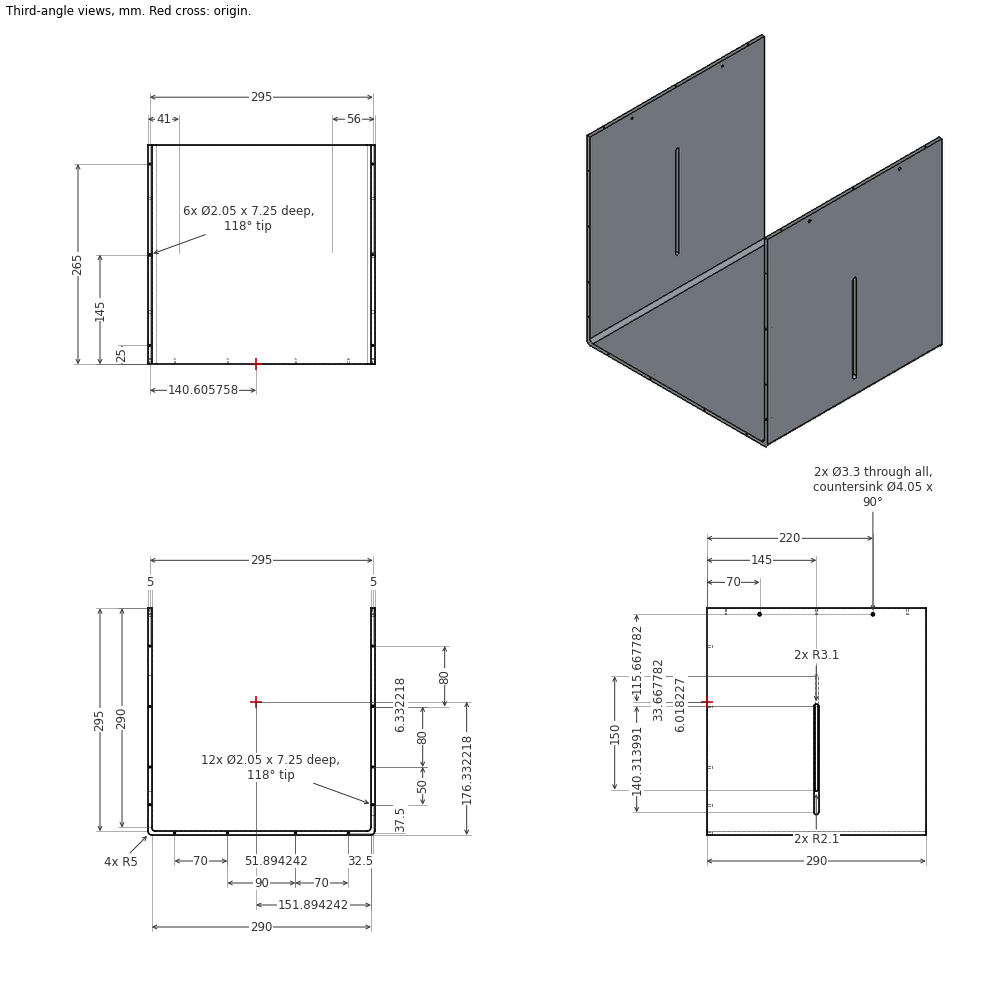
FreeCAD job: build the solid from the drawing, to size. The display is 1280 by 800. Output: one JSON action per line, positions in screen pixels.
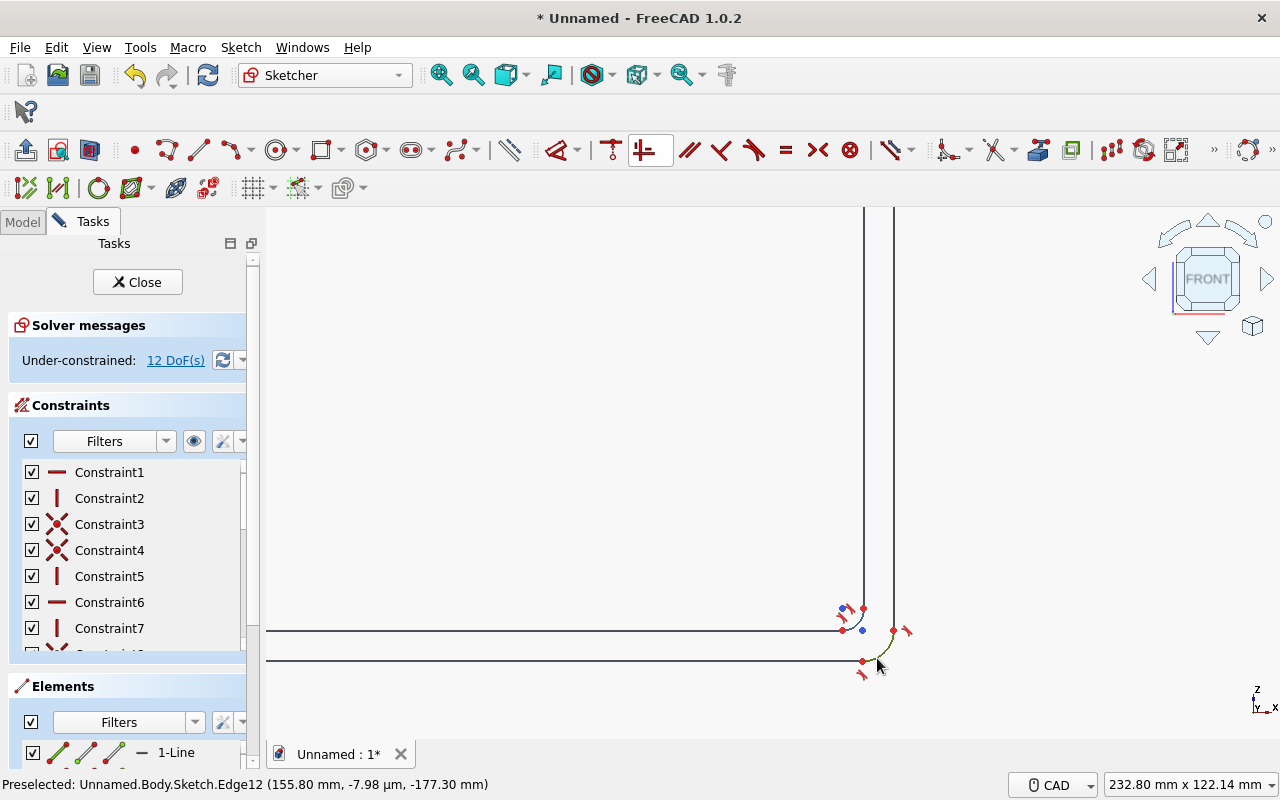
{"action": "left_click", "coordinate": [786, 150]}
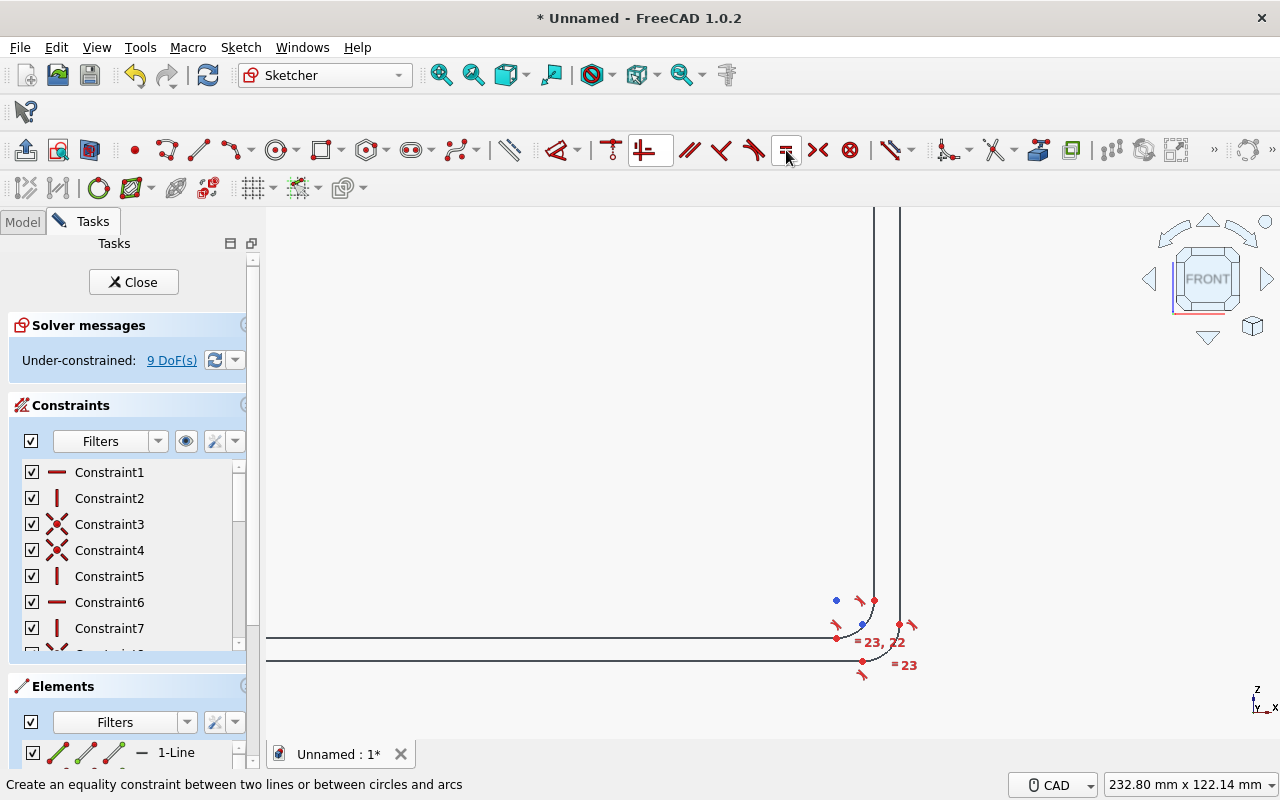
{"action": "left_click", "coordinate": [556, 150]}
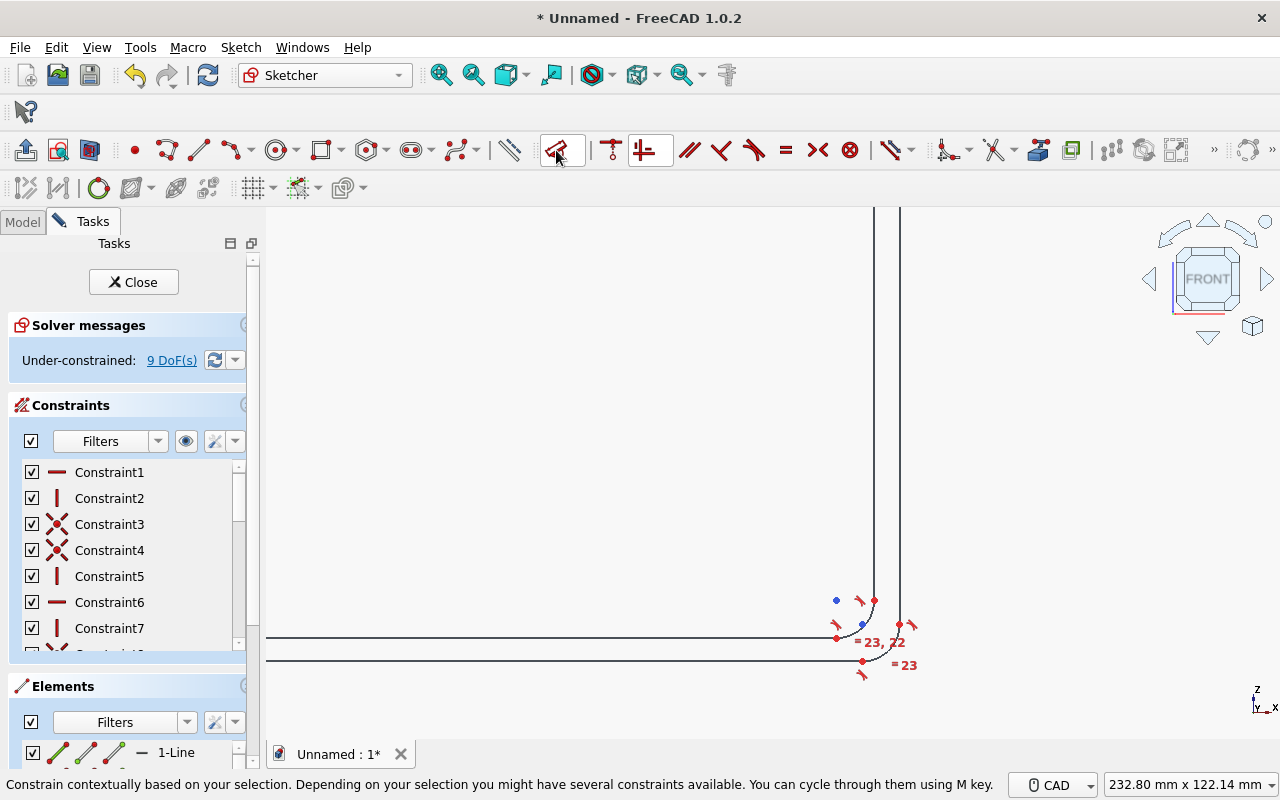
{"action": "scroll", "coordinate": [859, 628], "scroll_direction": "down", "scroll_amount": 7}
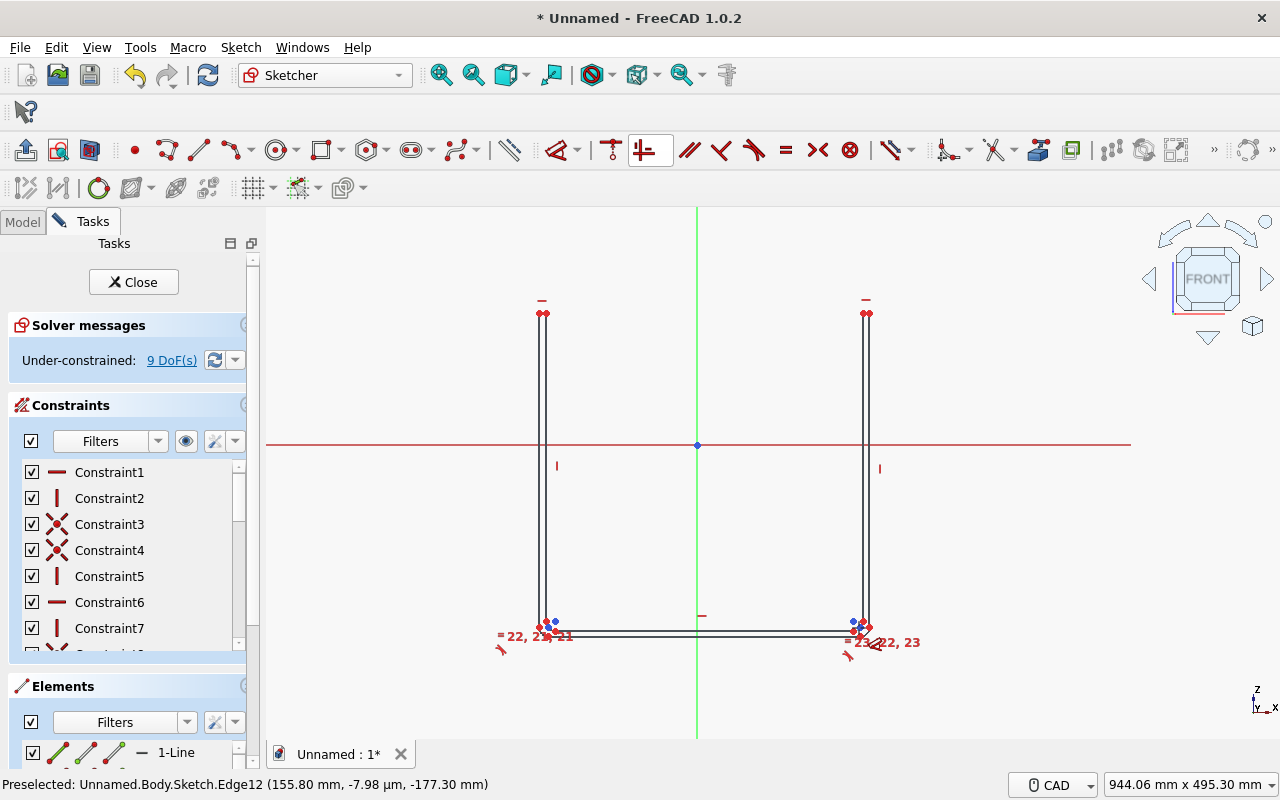
{"action": "scroll", "coordinate": [540, 632], "scroll_direction": "up", "scroll_amount": 11}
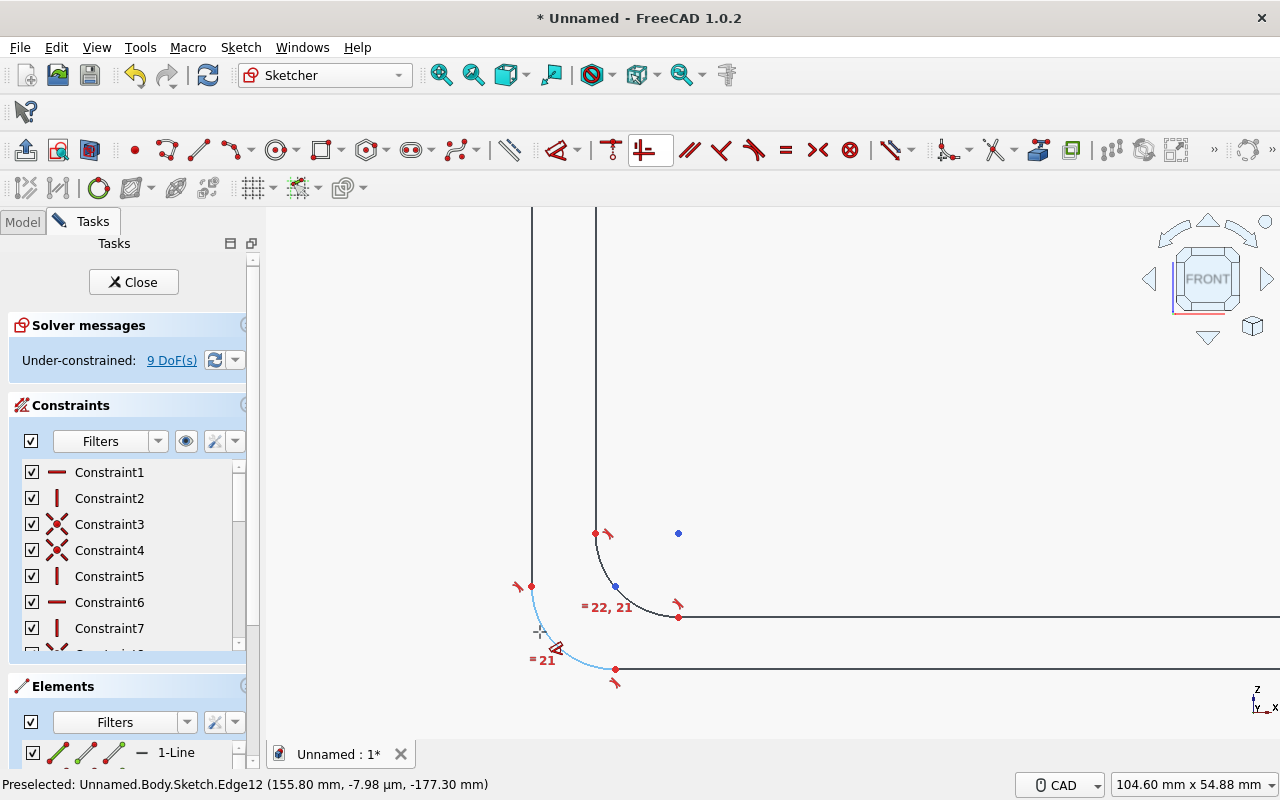
{"action": "left_click", "coordinate": [541, 624]}
{"action": "left_click", "coordinate": [513, 639]}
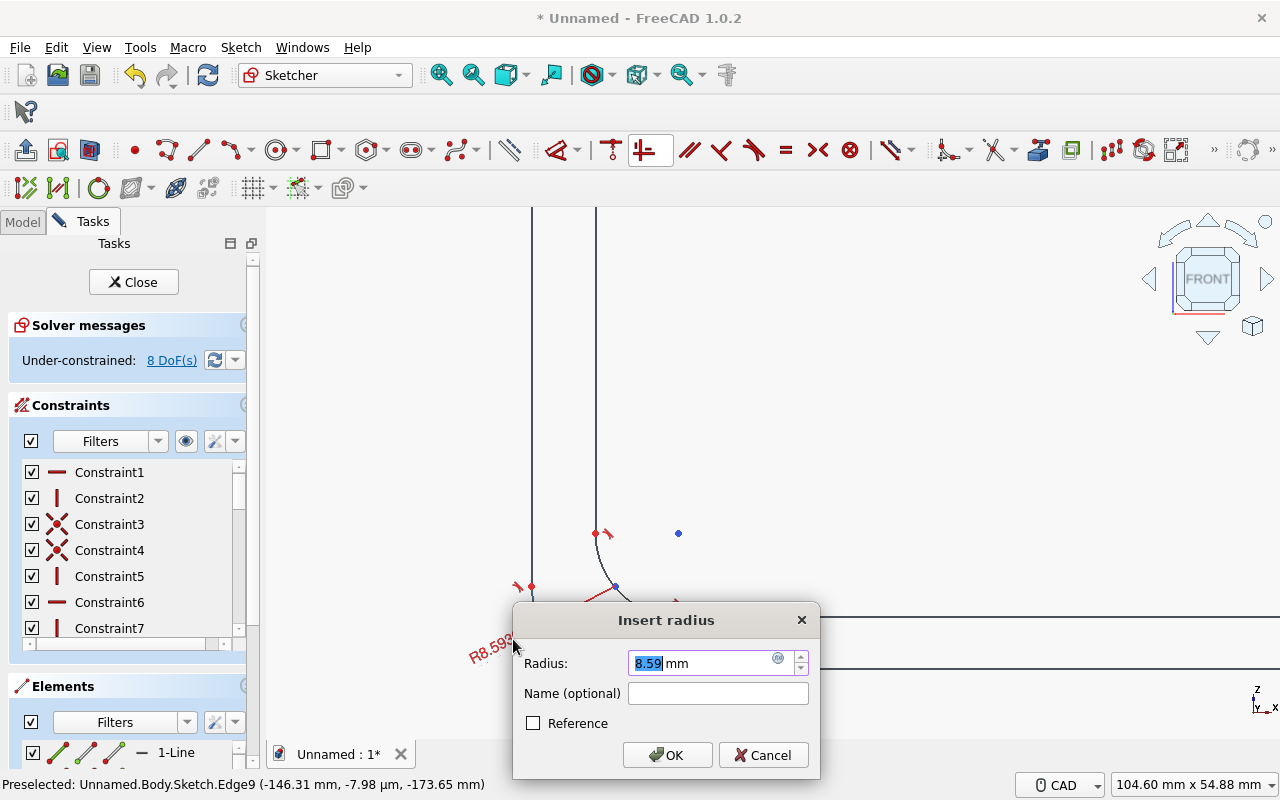
{"action": "type", "text": "5"}
{"action": "key", "text": "Return"}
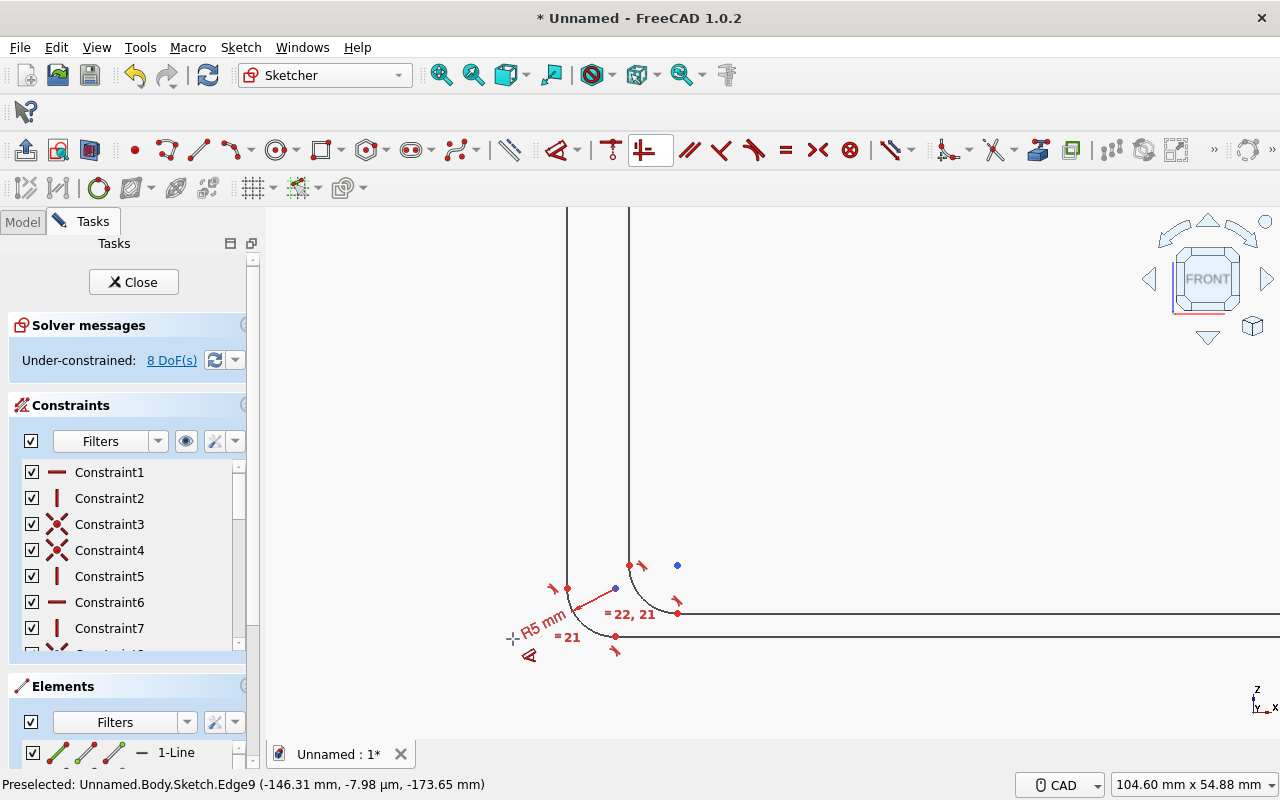
{"action": "scroll", "coordinate": [540, 632], "scroll_direction": "down", "scroll_amount": 11}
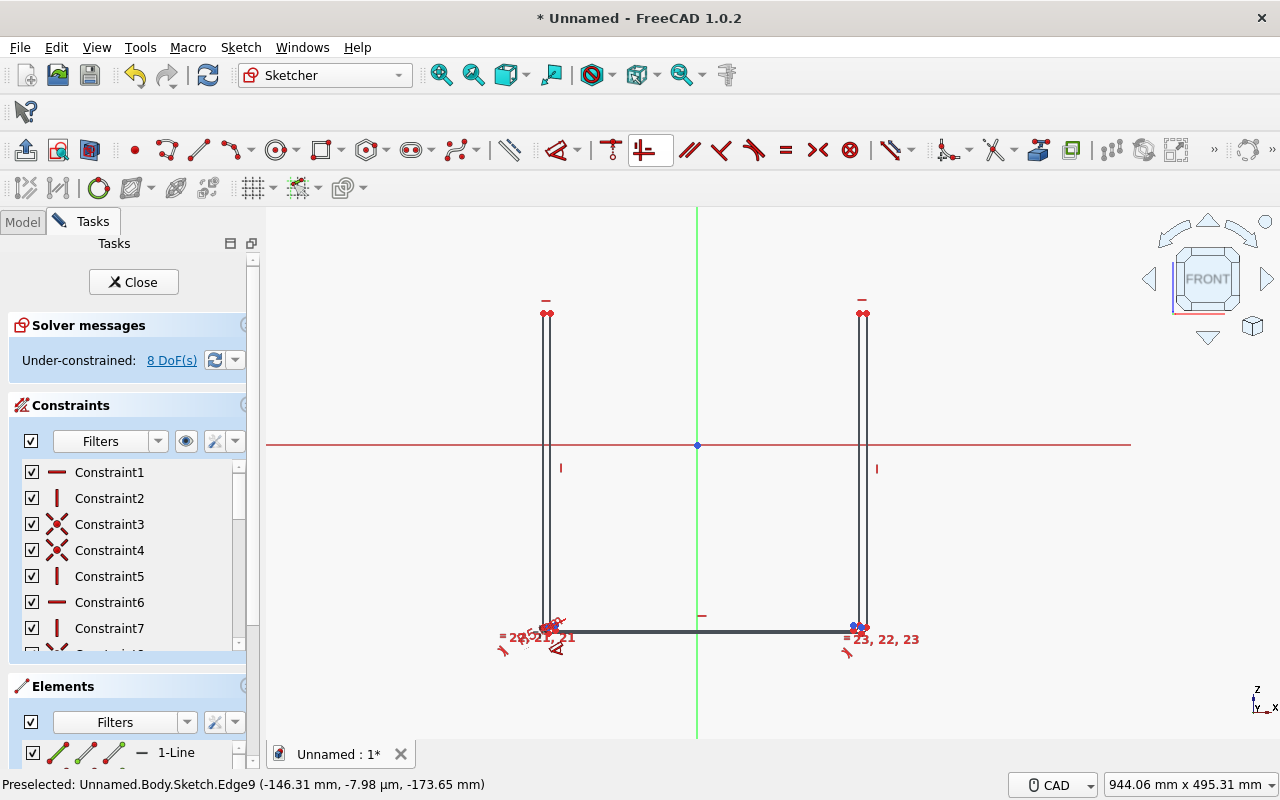
{"action": "scroll", "coordinate": [545, 314], "scroll_direction": "up", "scroll_amount": 11}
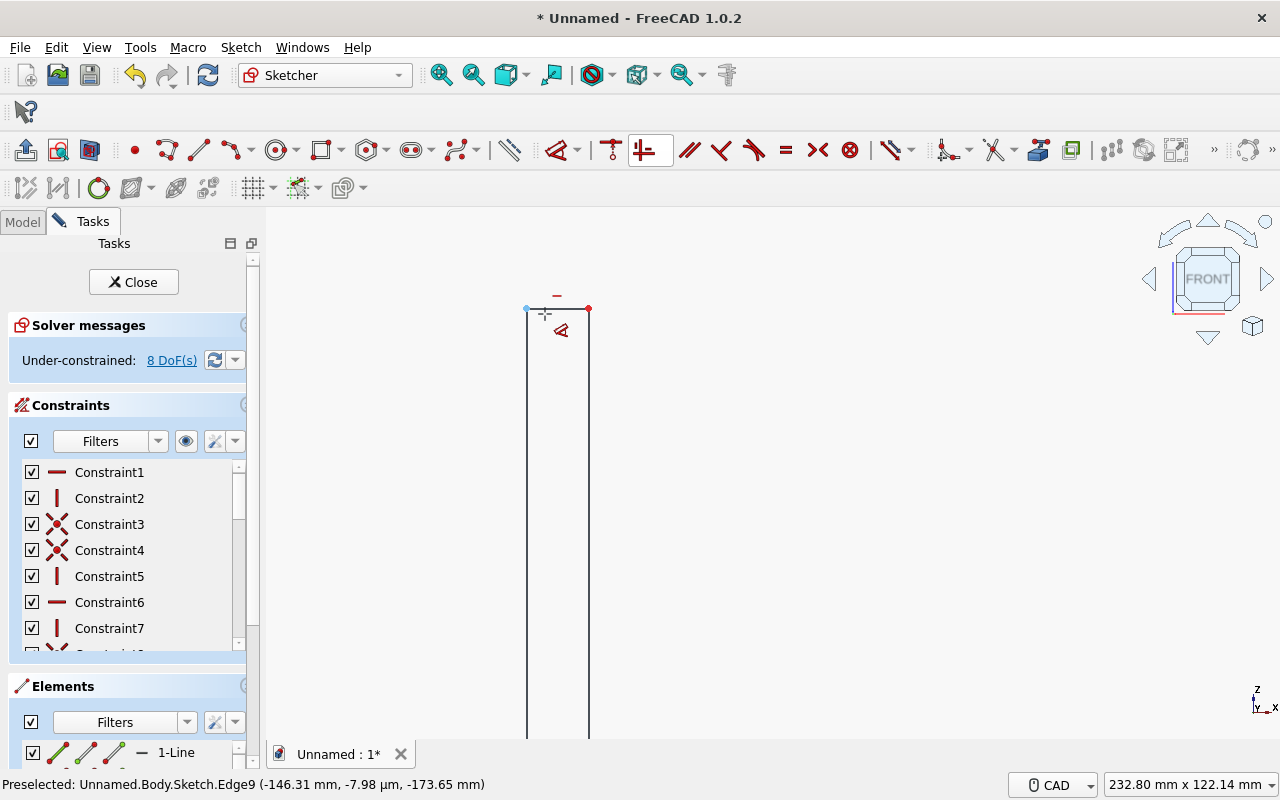
{"action": "left_click", "coordinate": [546, 309]}
{"action": "left_click", "coordinate": [558, 275]}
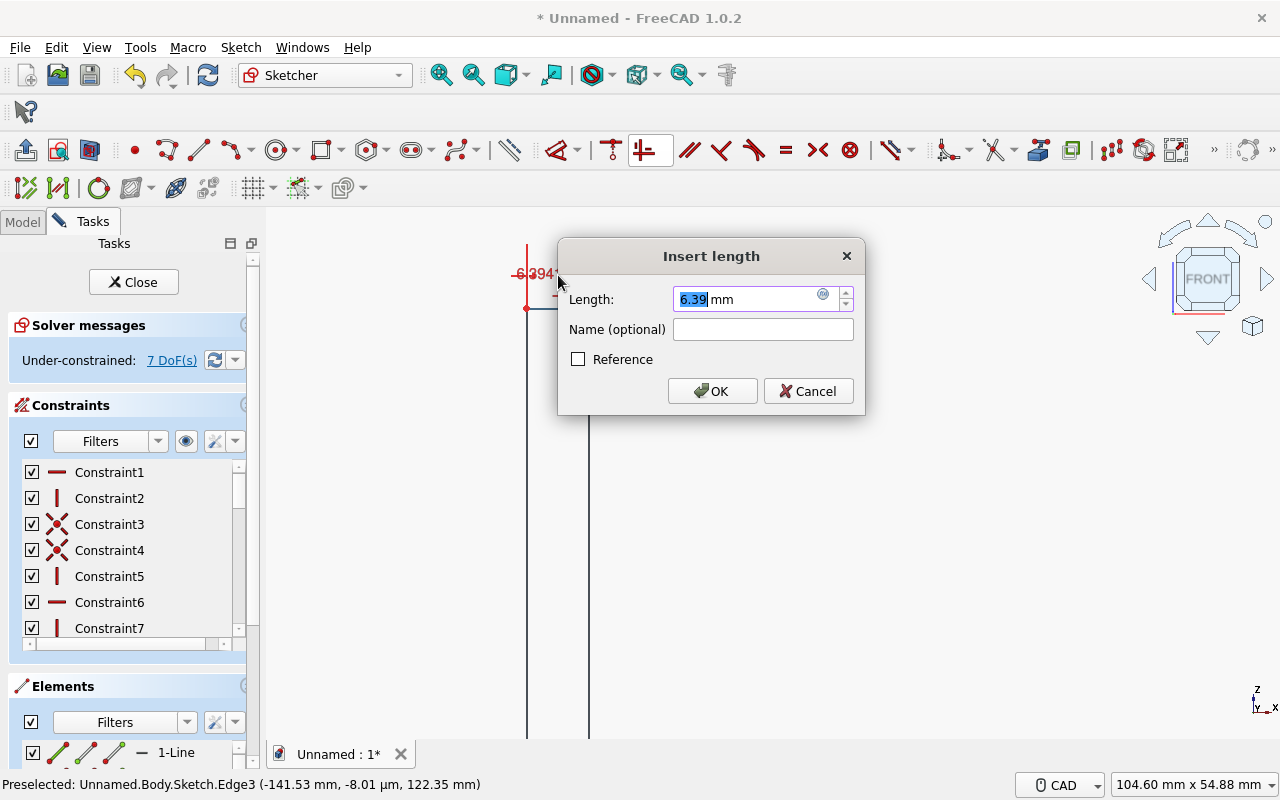
{"action": "type", "text": "5"}
{"action": "key", "text": "Return"}